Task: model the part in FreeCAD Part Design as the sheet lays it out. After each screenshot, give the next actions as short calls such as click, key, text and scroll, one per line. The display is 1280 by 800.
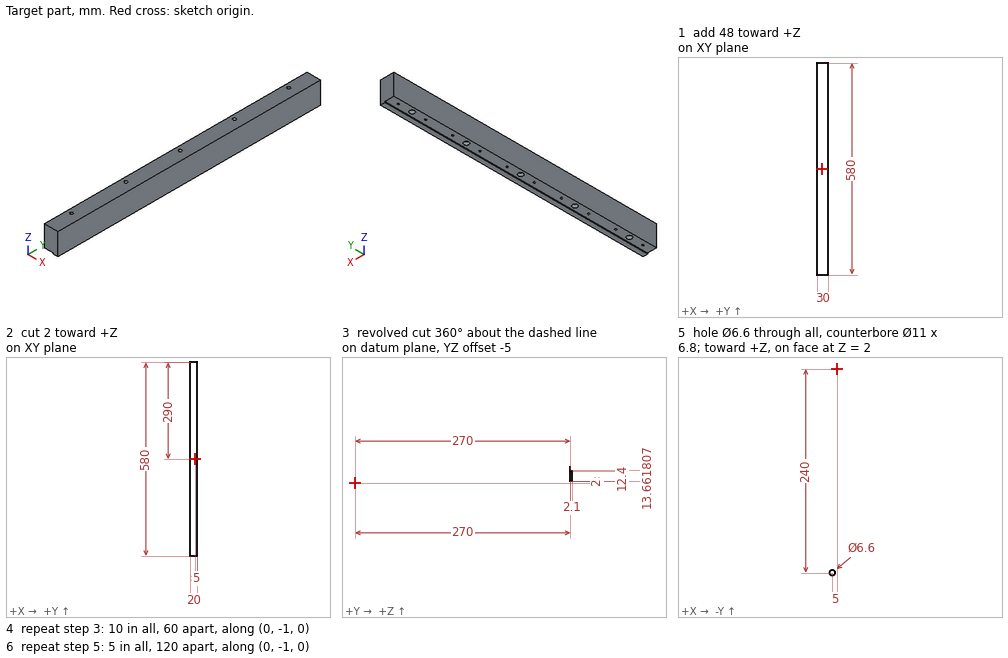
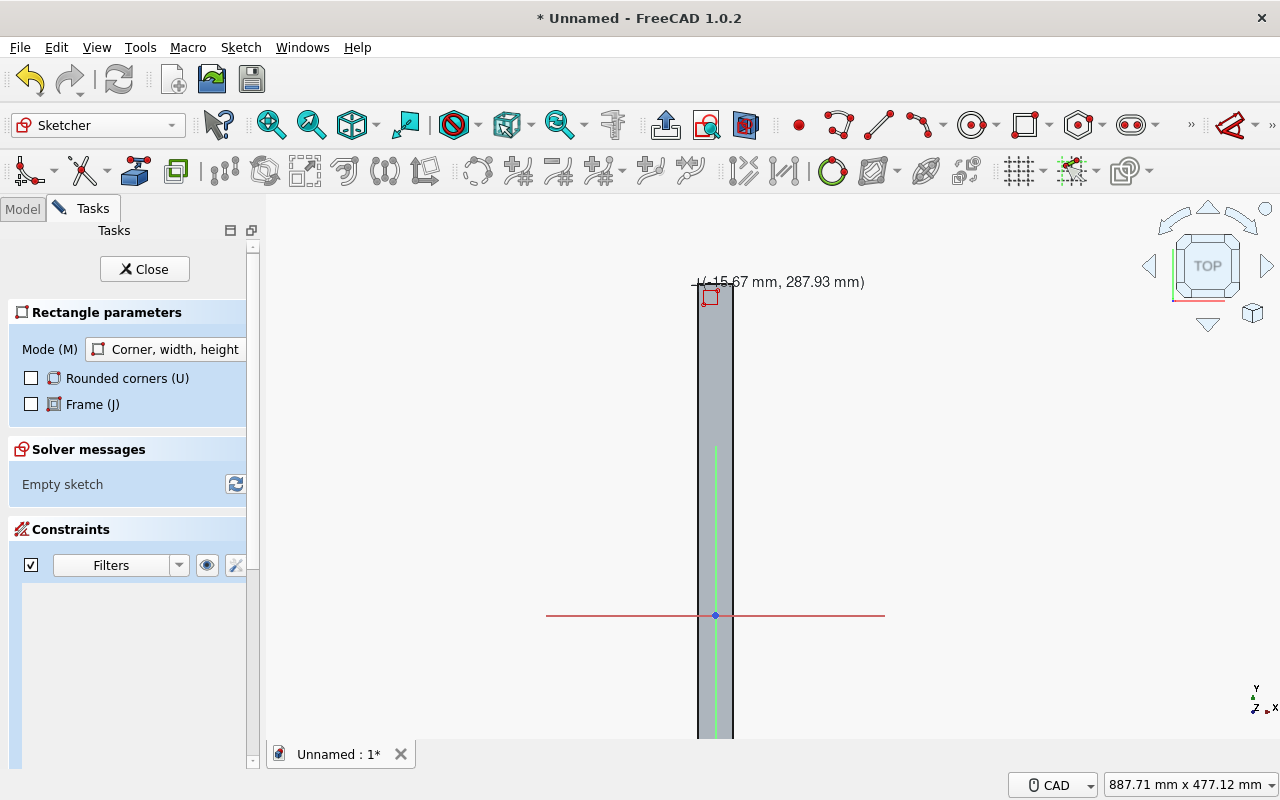
click(698, 284)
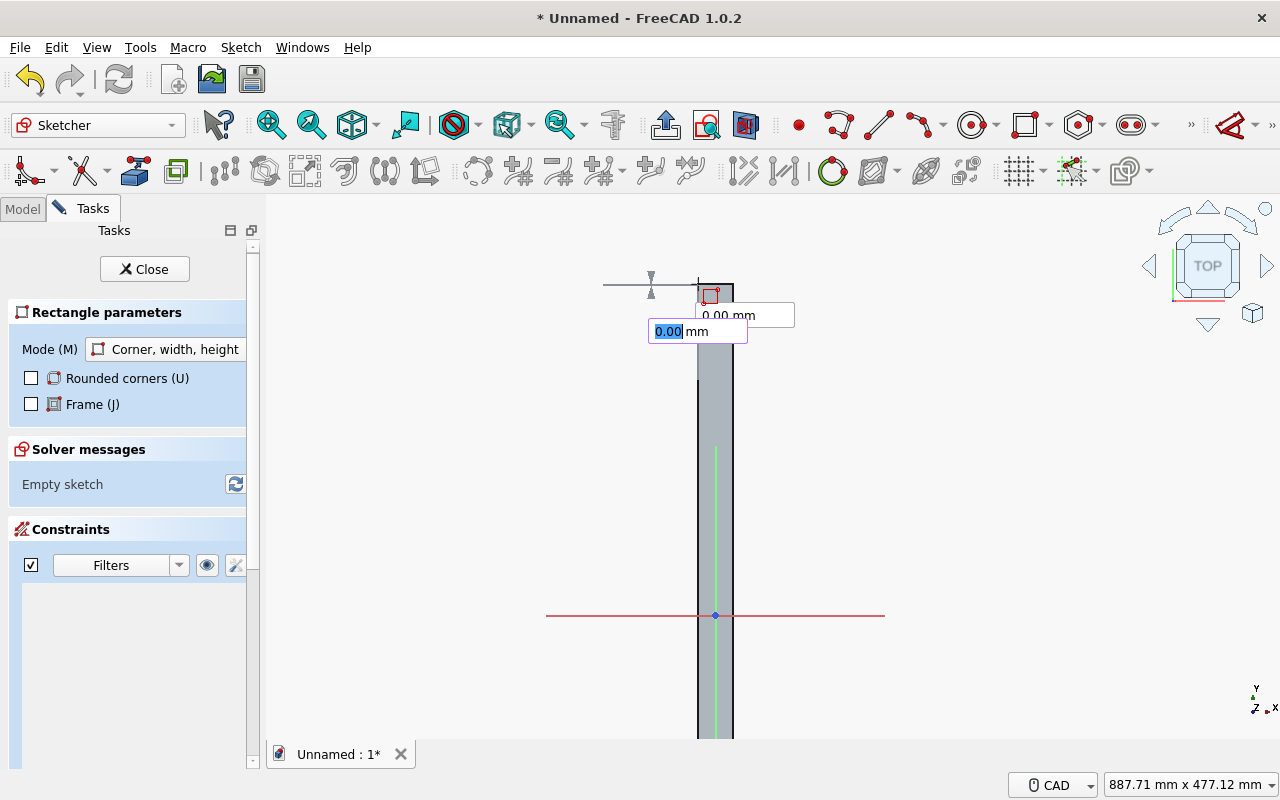
scroll(698, 285, down, 3)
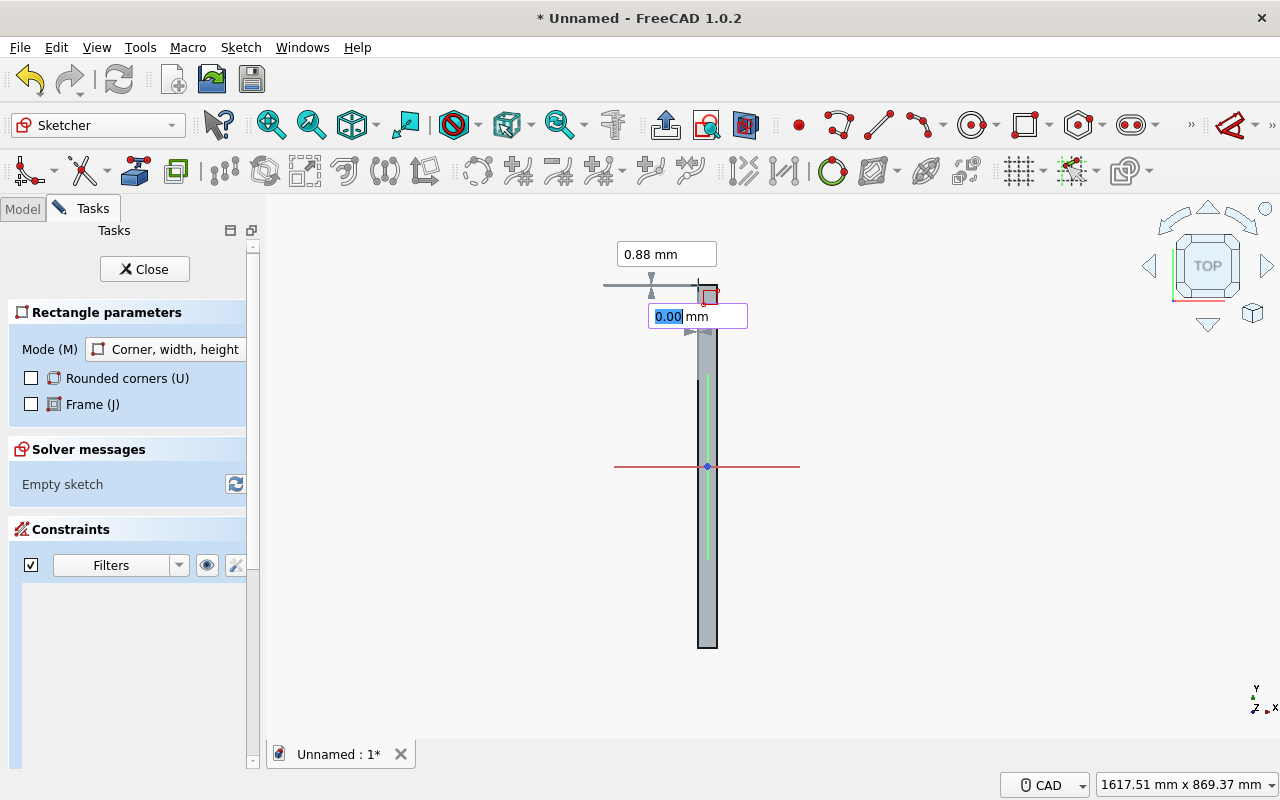
scroll(711, 648, up, 9)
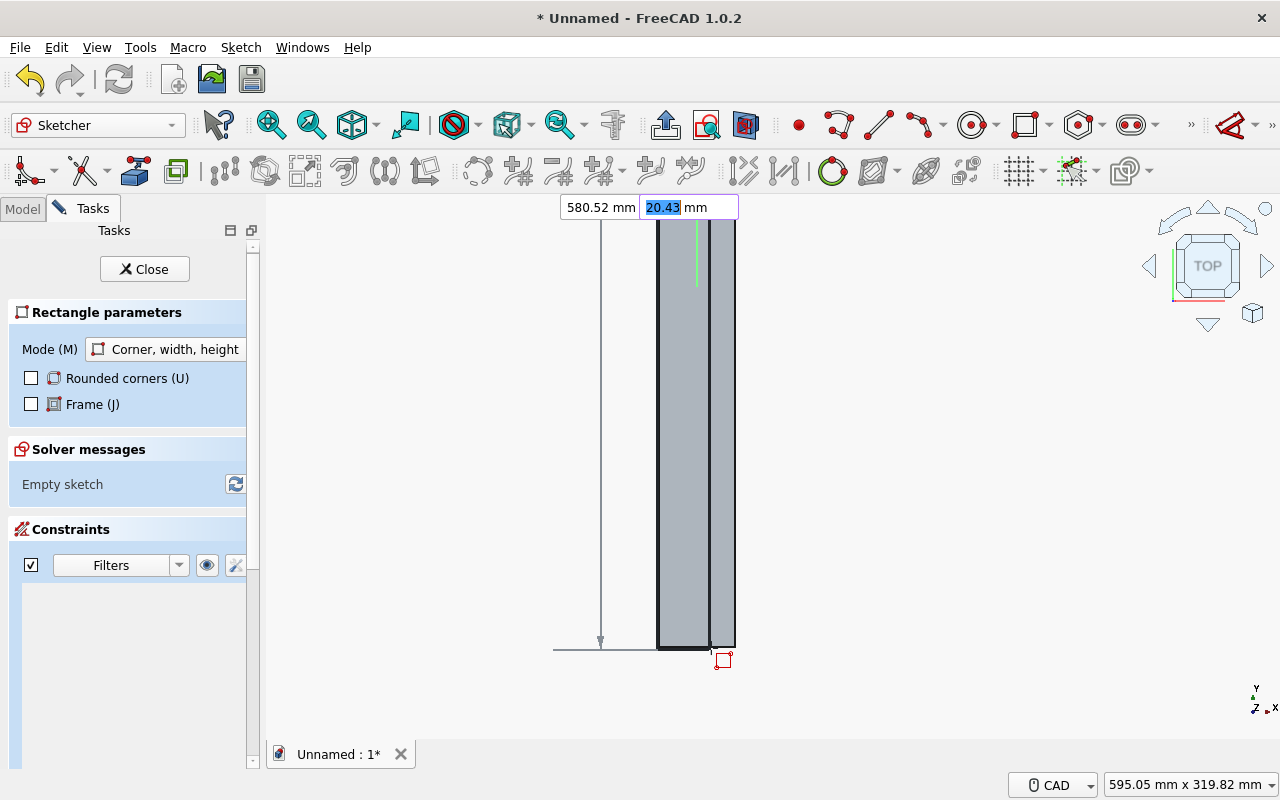
click(709, 646)
key(Escape)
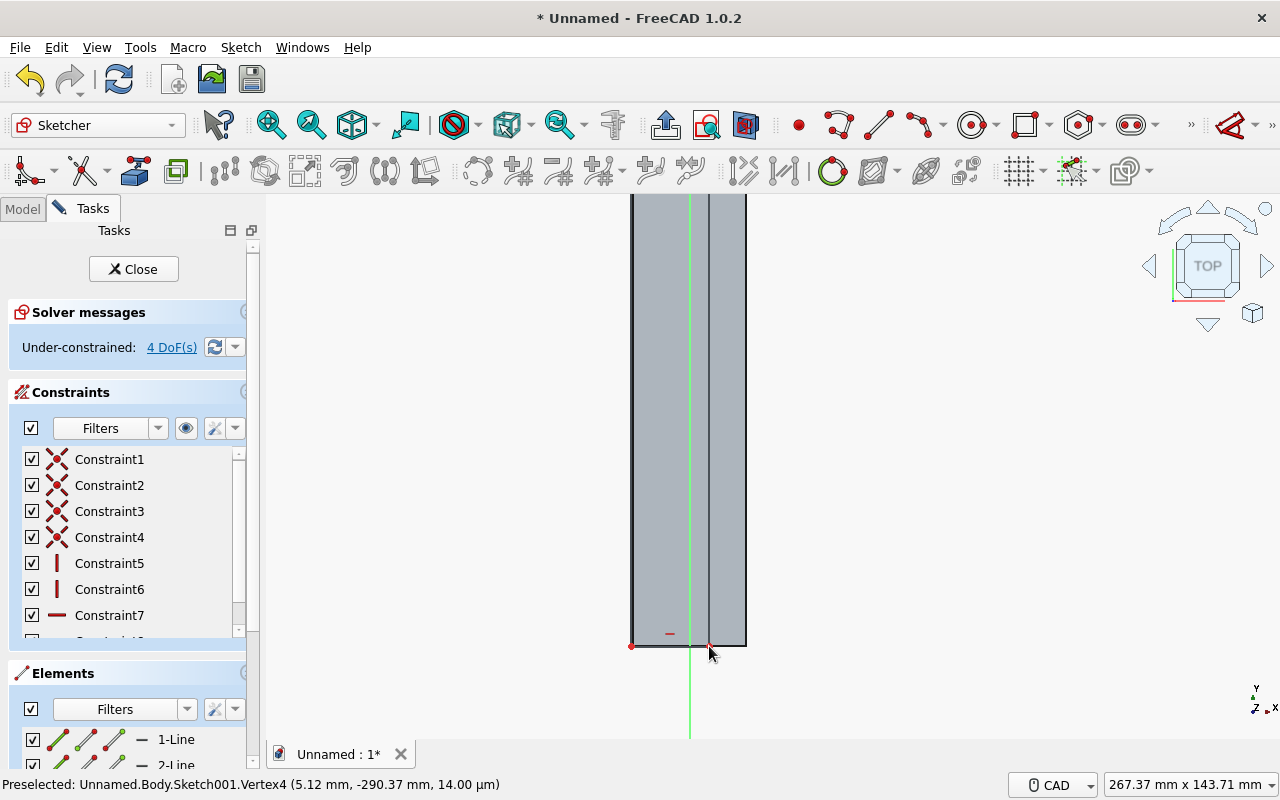
key(d)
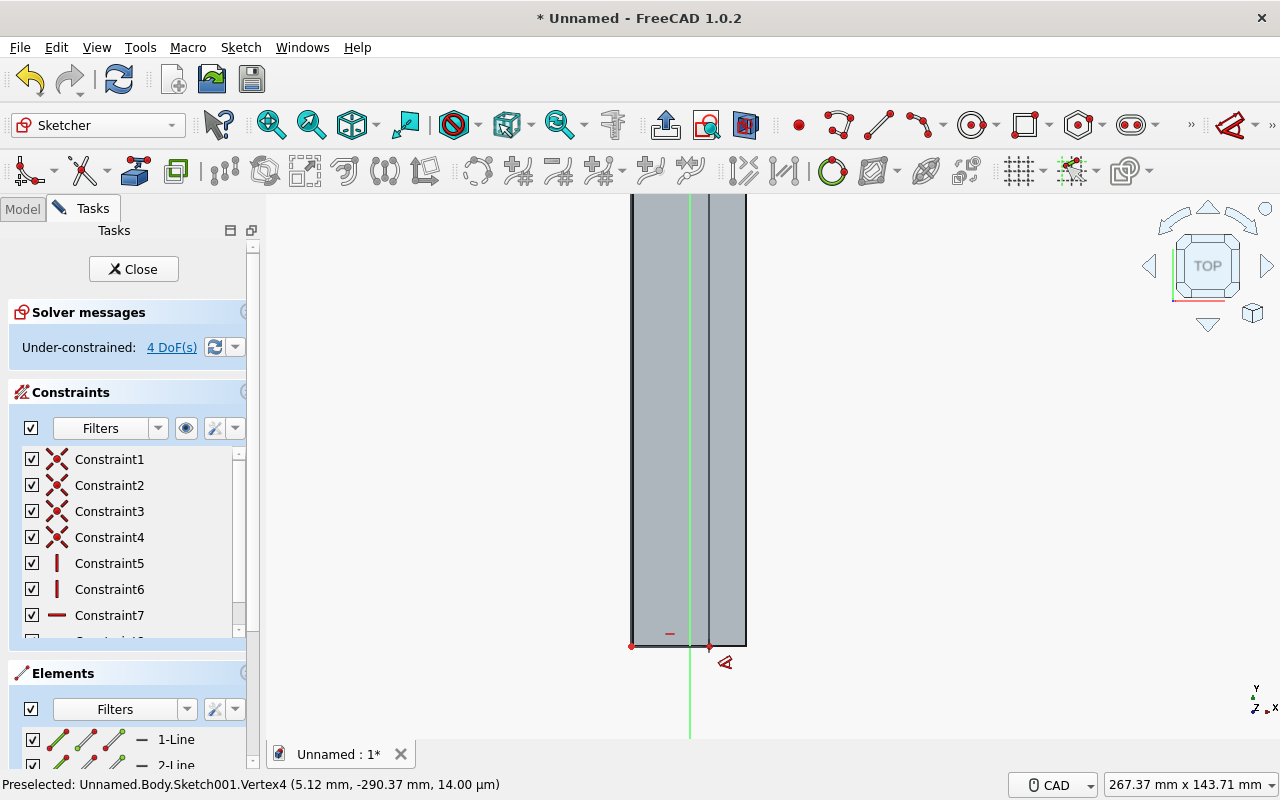
click(655, 647)
click(670, 681)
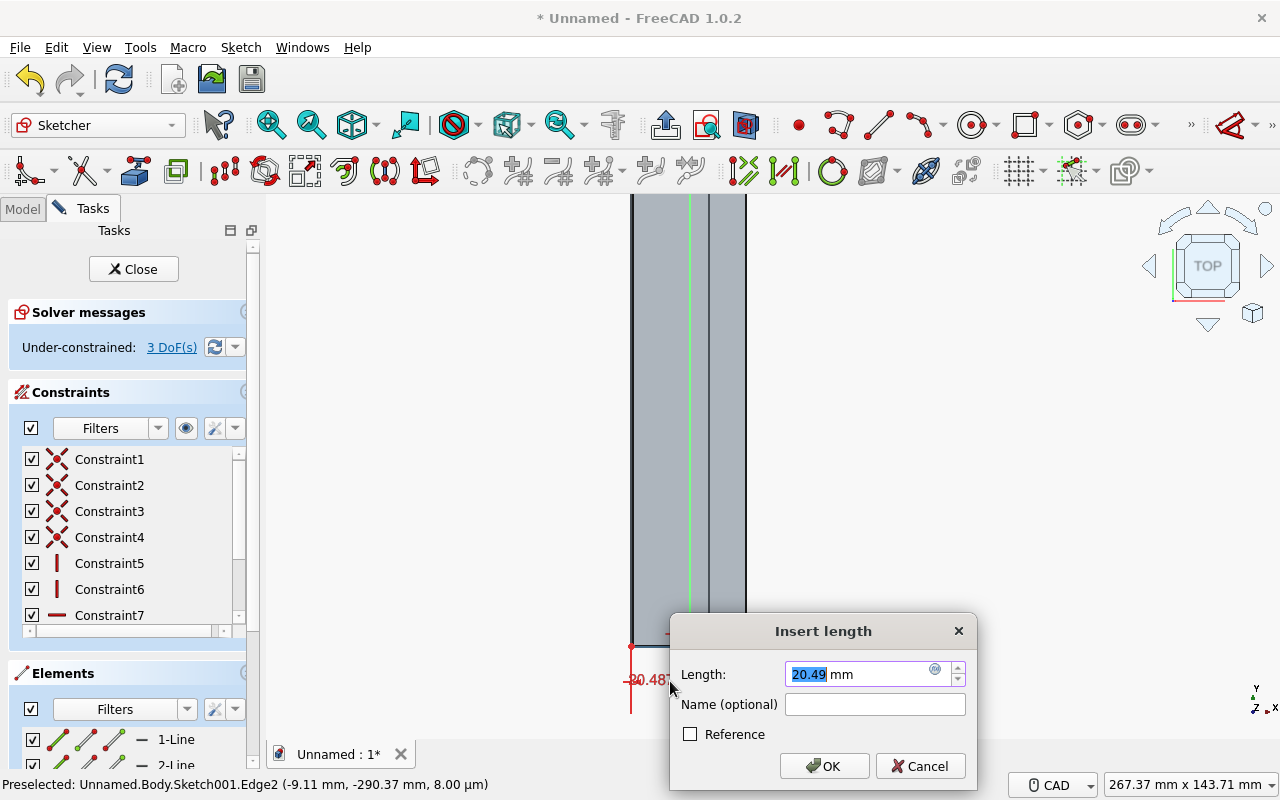
text(20)
key(Return)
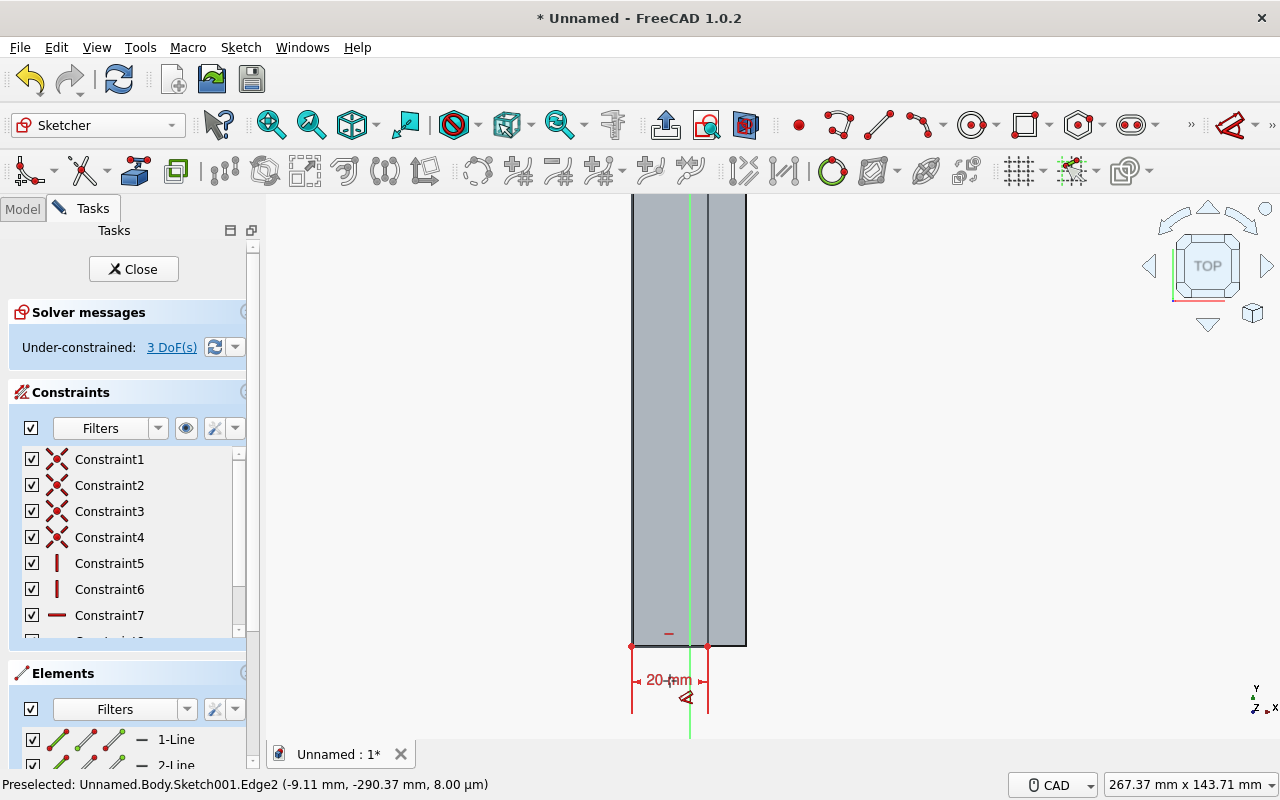
scroll(708, 647, up, 4)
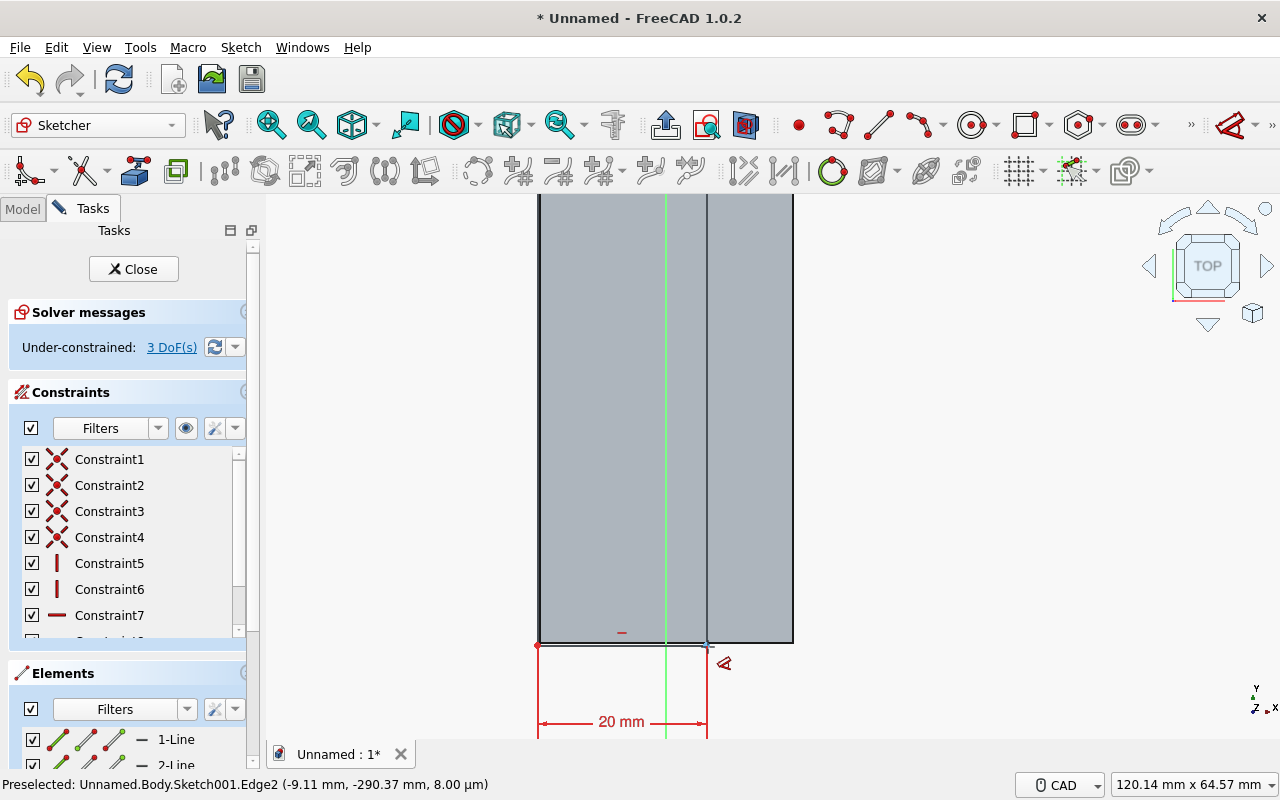
click(707, 646)
click(687, 680)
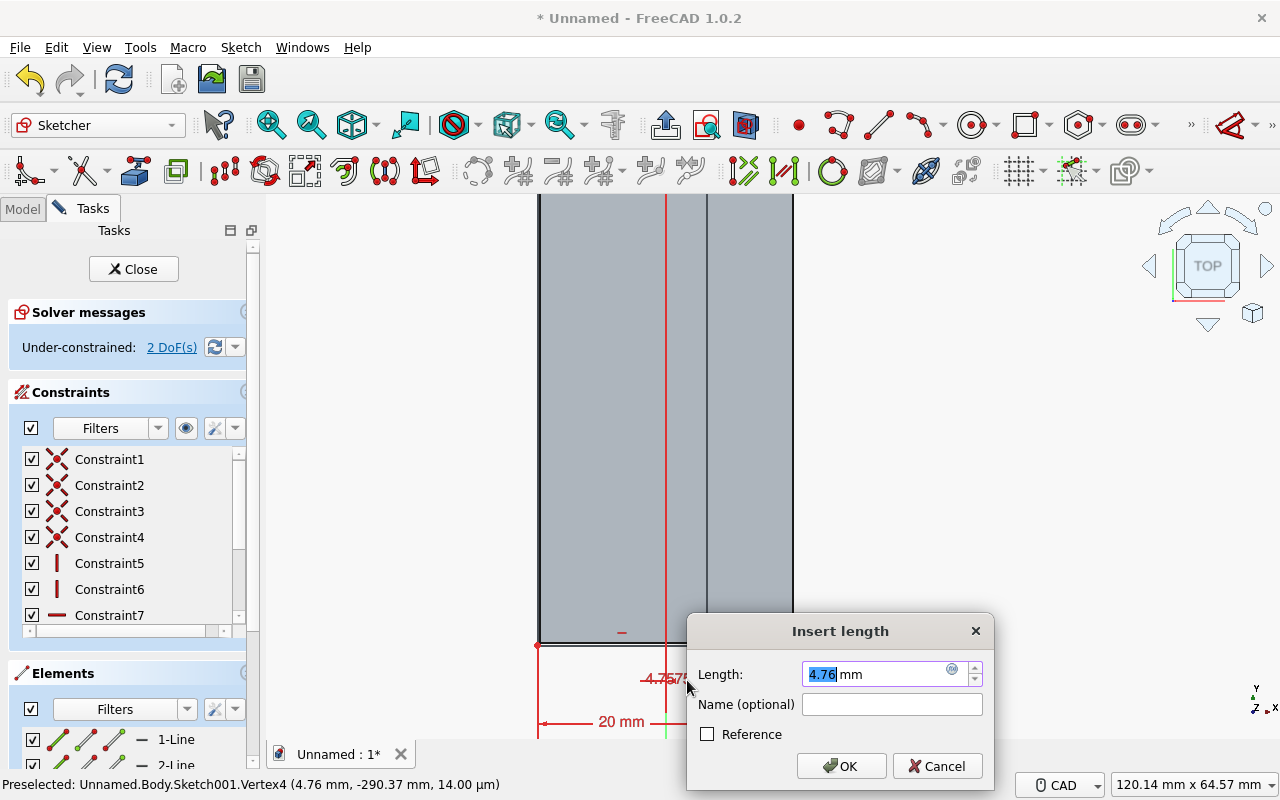
text(5)
key(Return)